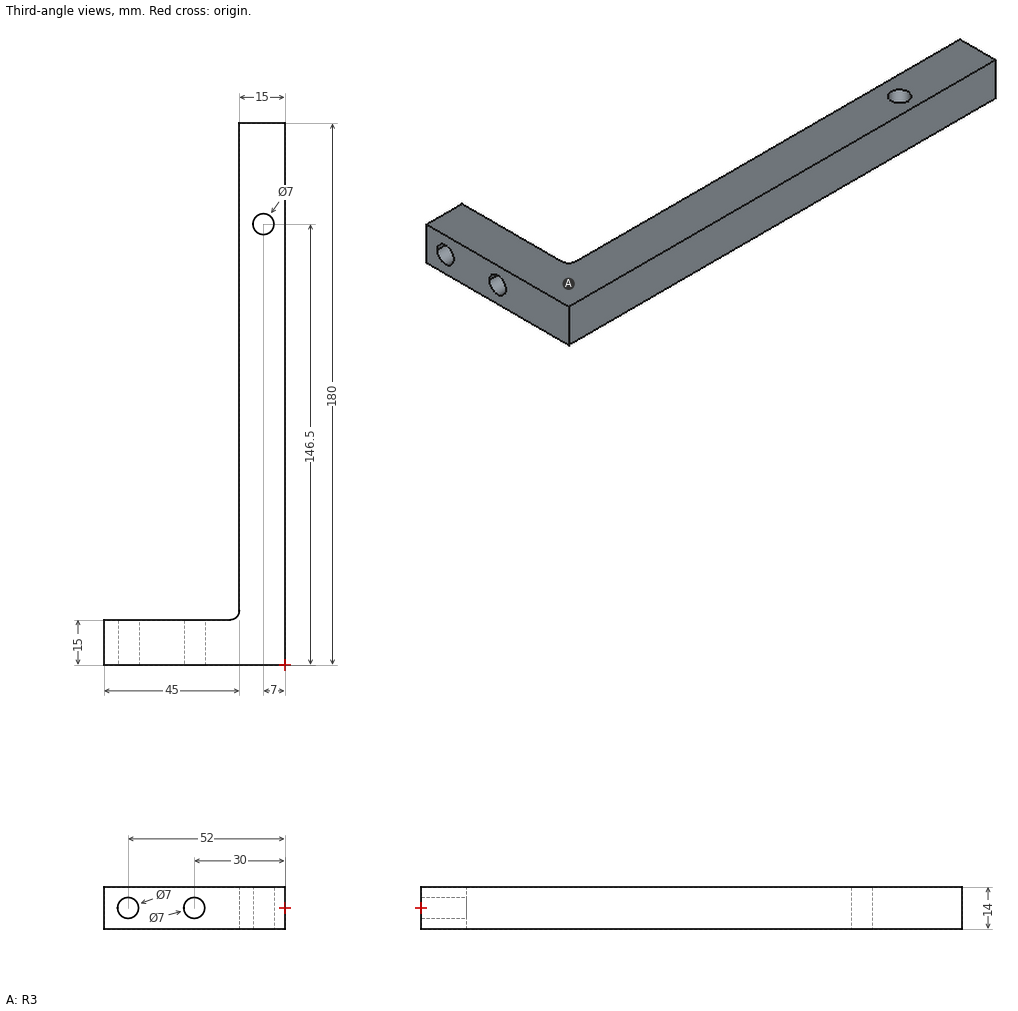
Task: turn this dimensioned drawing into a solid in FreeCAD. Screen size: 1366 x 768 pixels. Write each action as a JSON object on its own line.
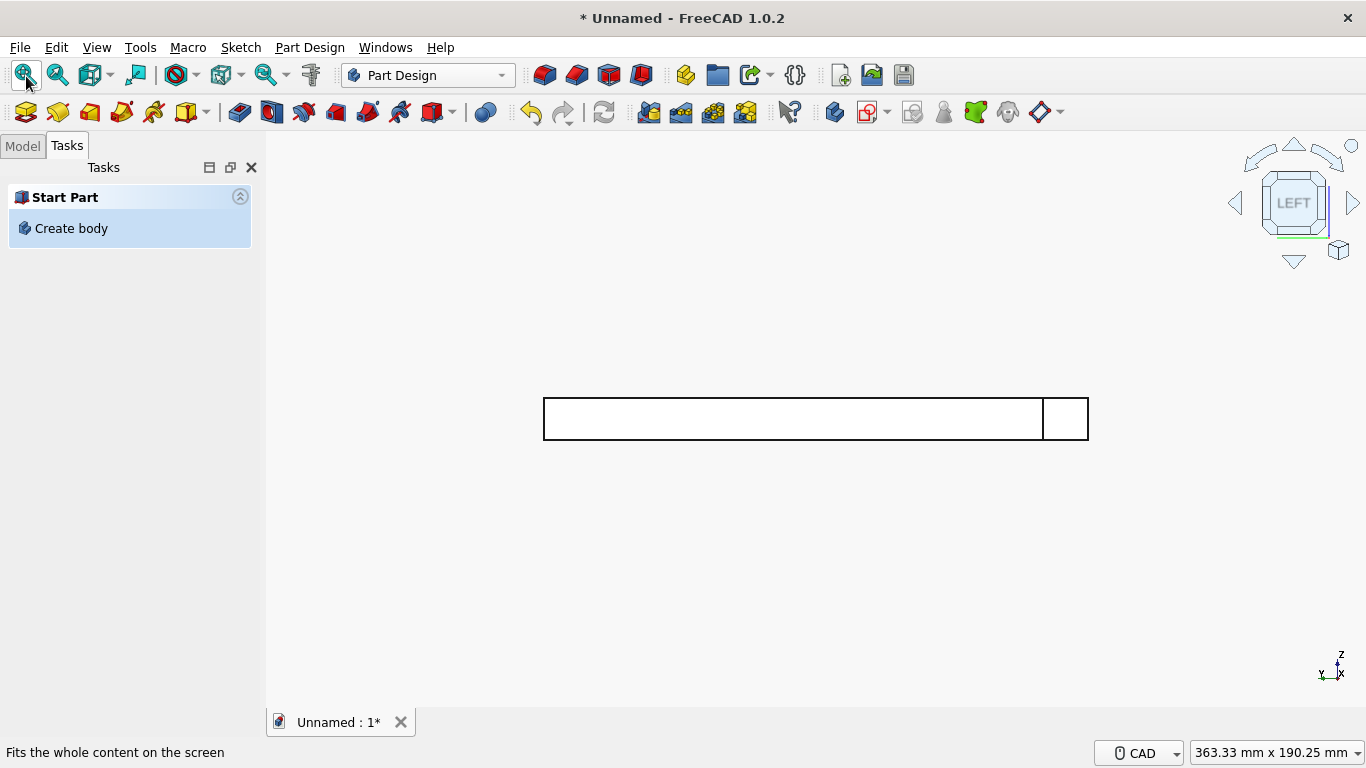
{"action": "key", "text": "v 3"}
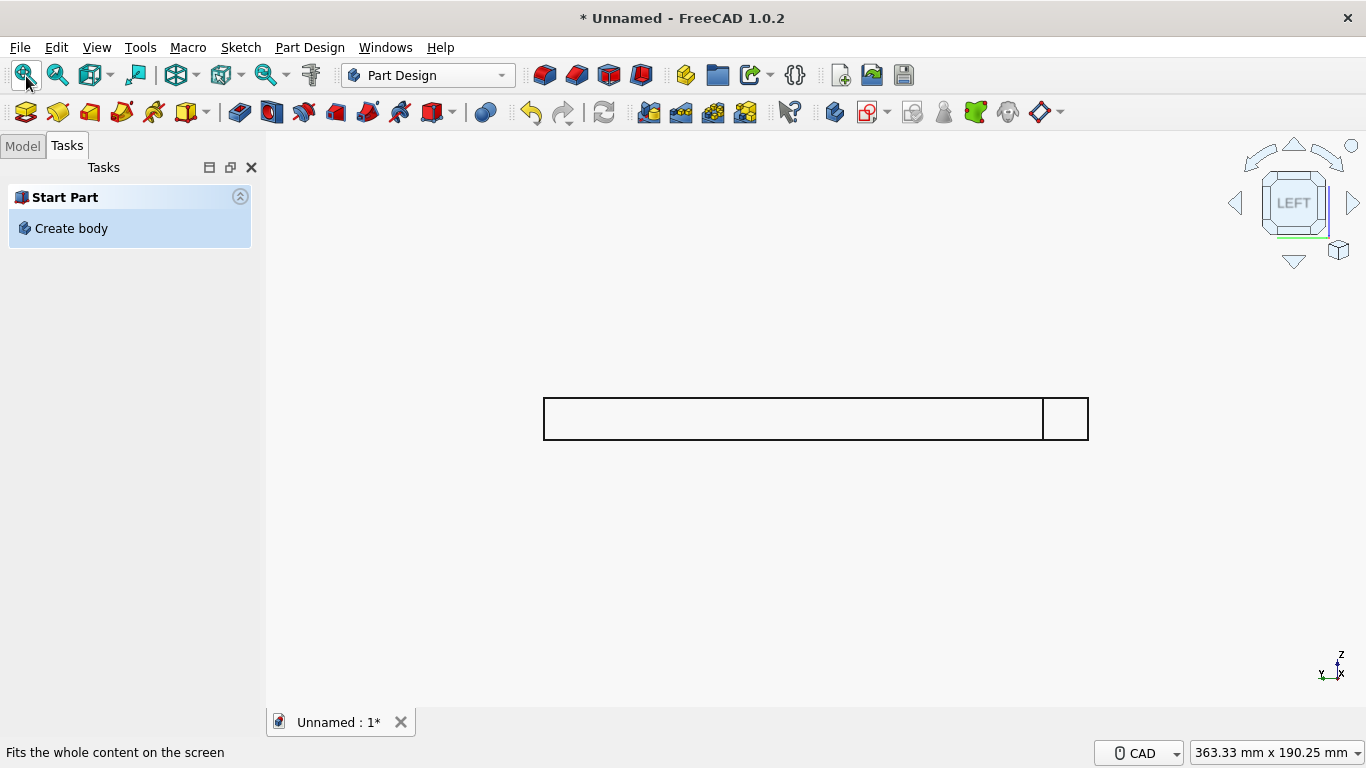
{"action": "key", "text": "0"}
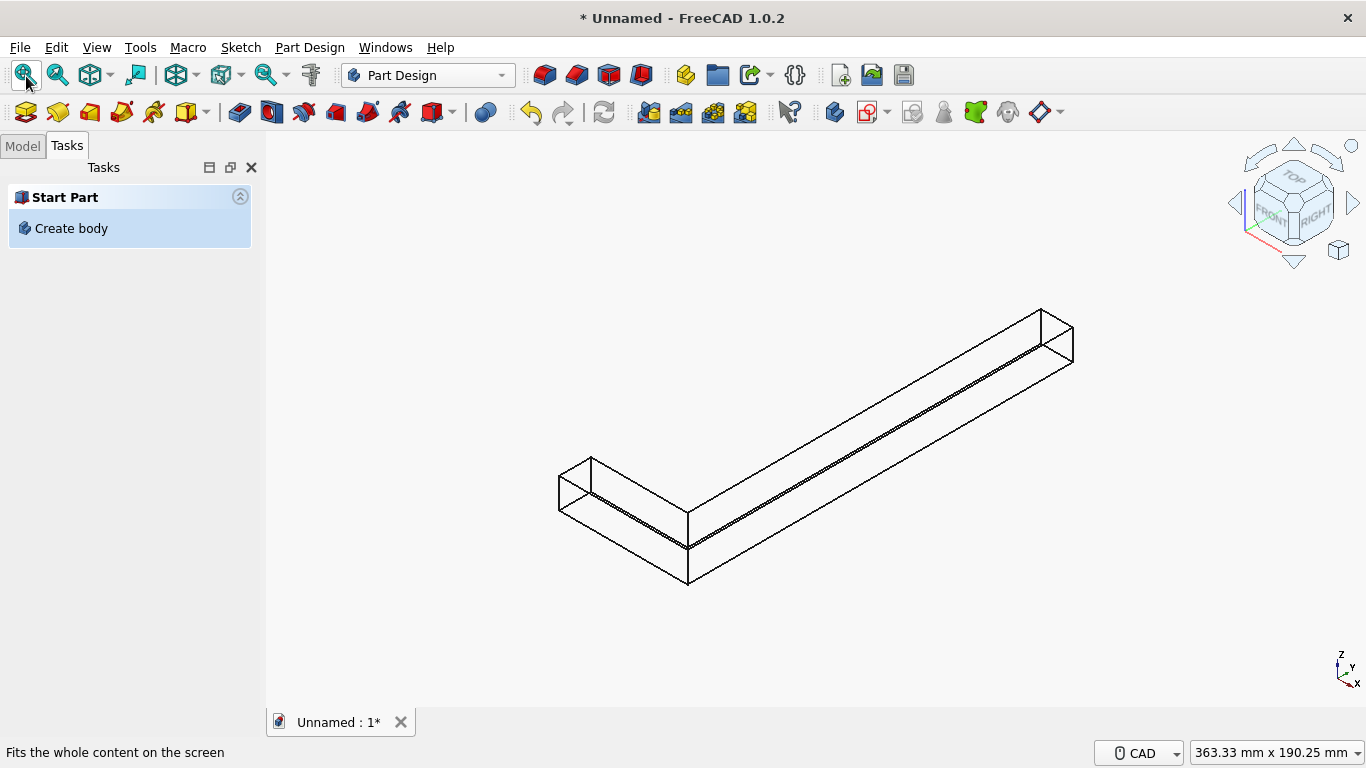
{"action": "left_click", "coordinate": [688, 529]}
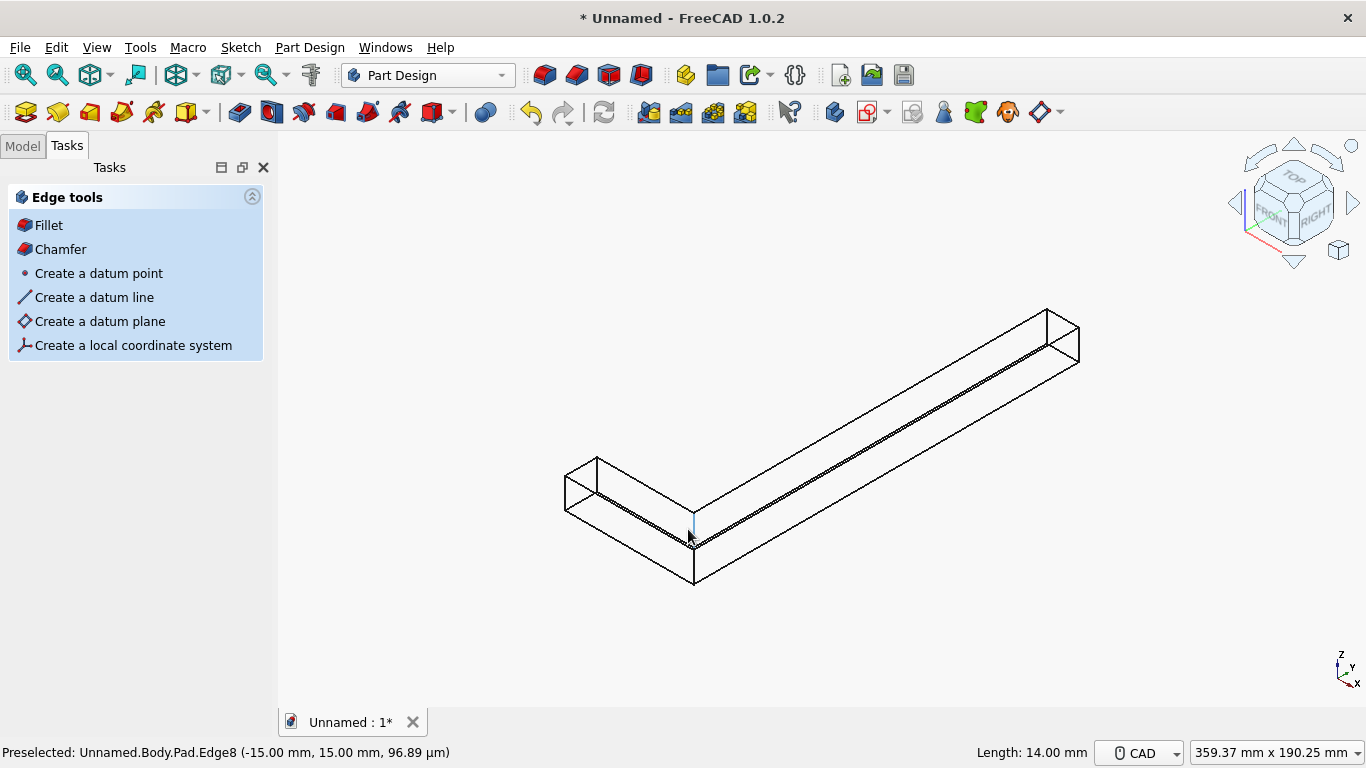
{"action": "key", "text": "v 1"}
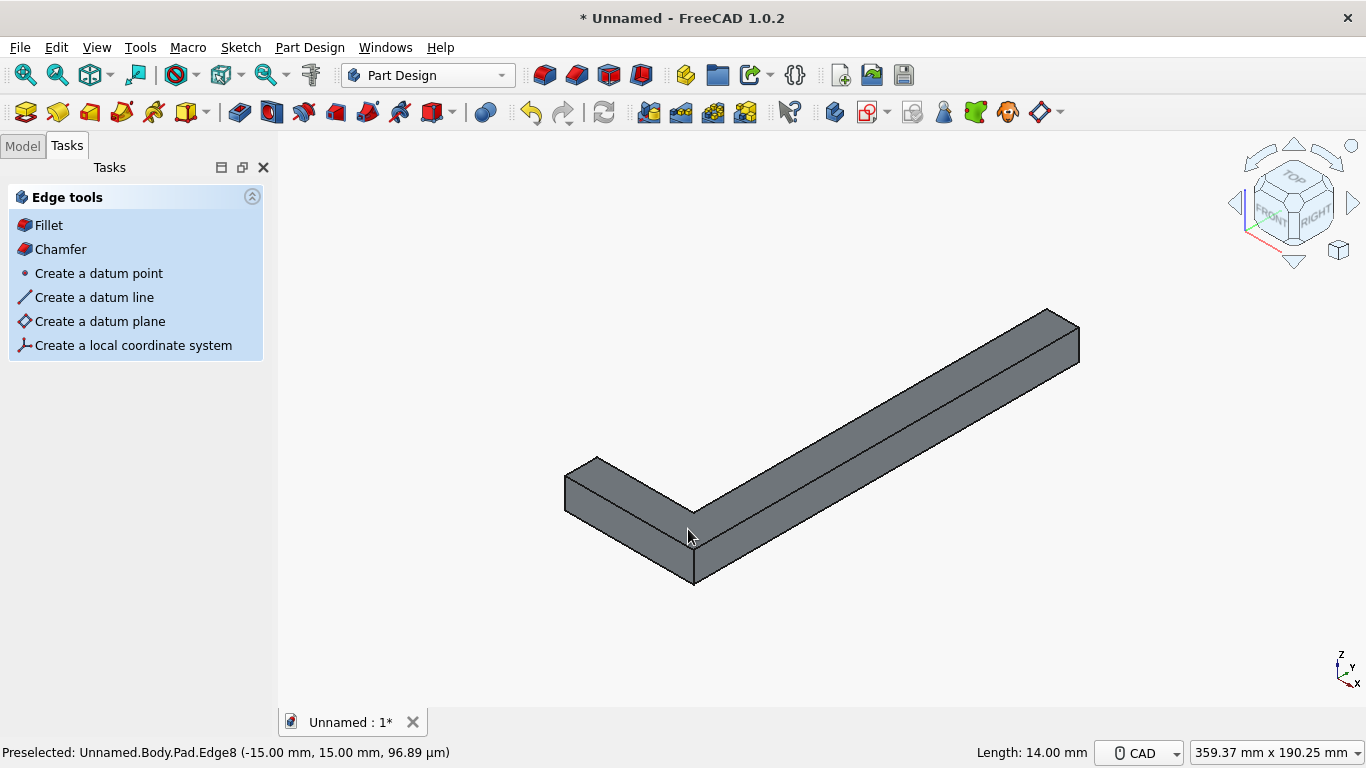
{"action": "left_click", "coordinate": [546, 76]}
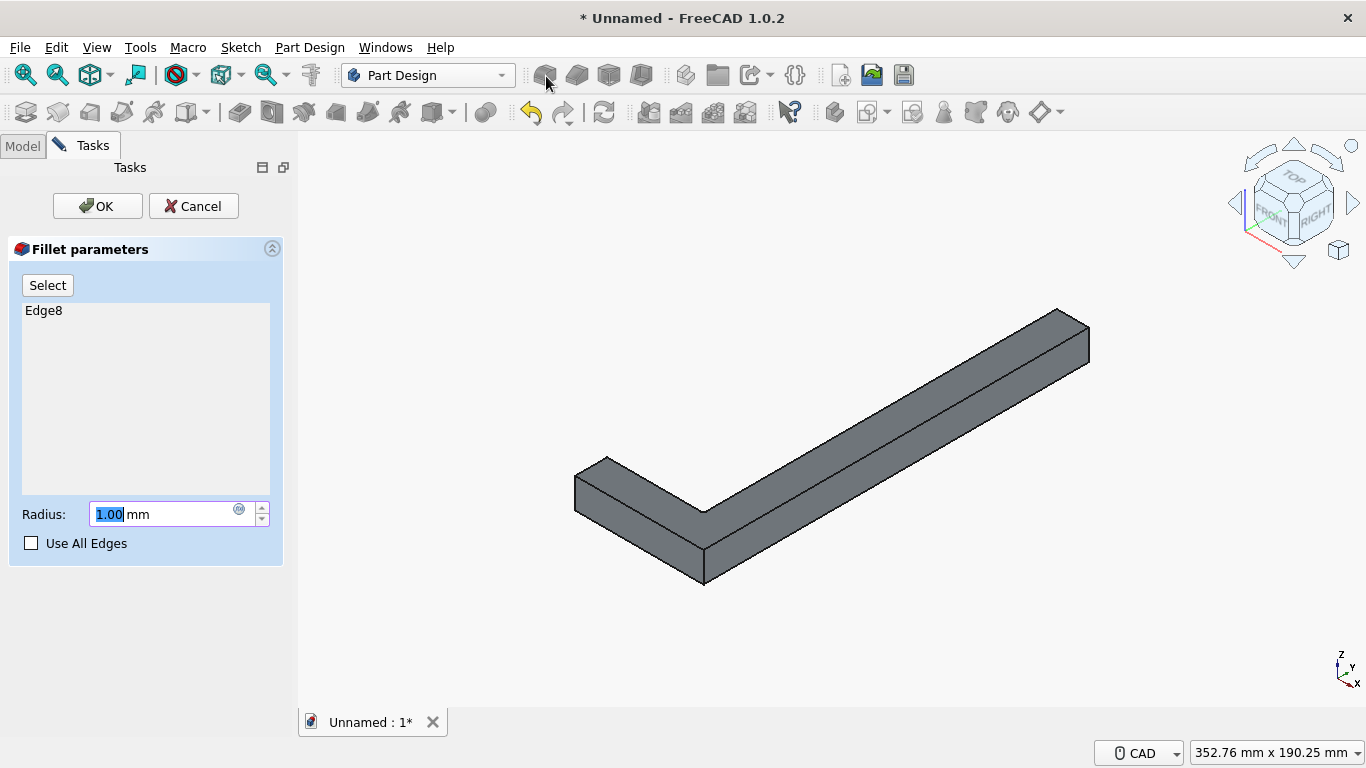
{"action": "type", "text": "3"}
{"action": "key", "text": "Tab"}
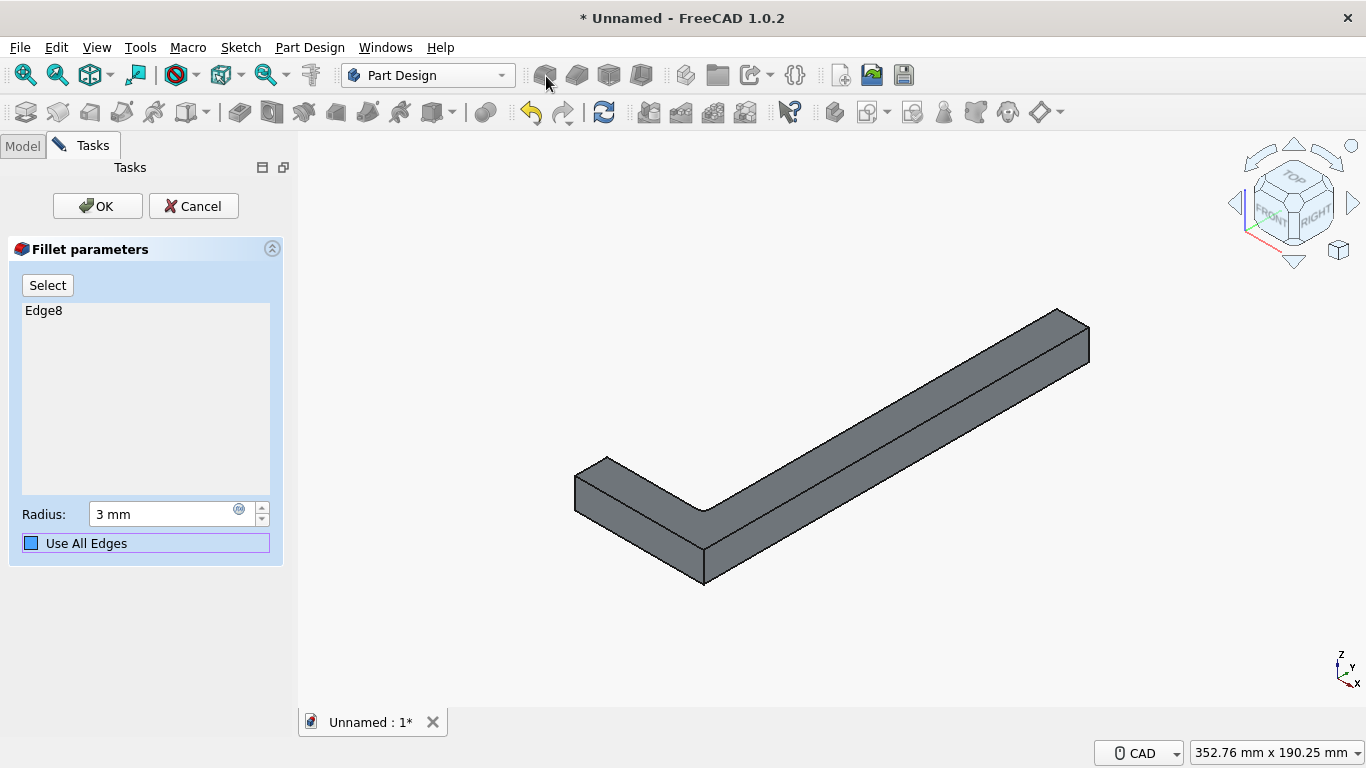
{"action": "left_click", "coordinate": [98, 206]}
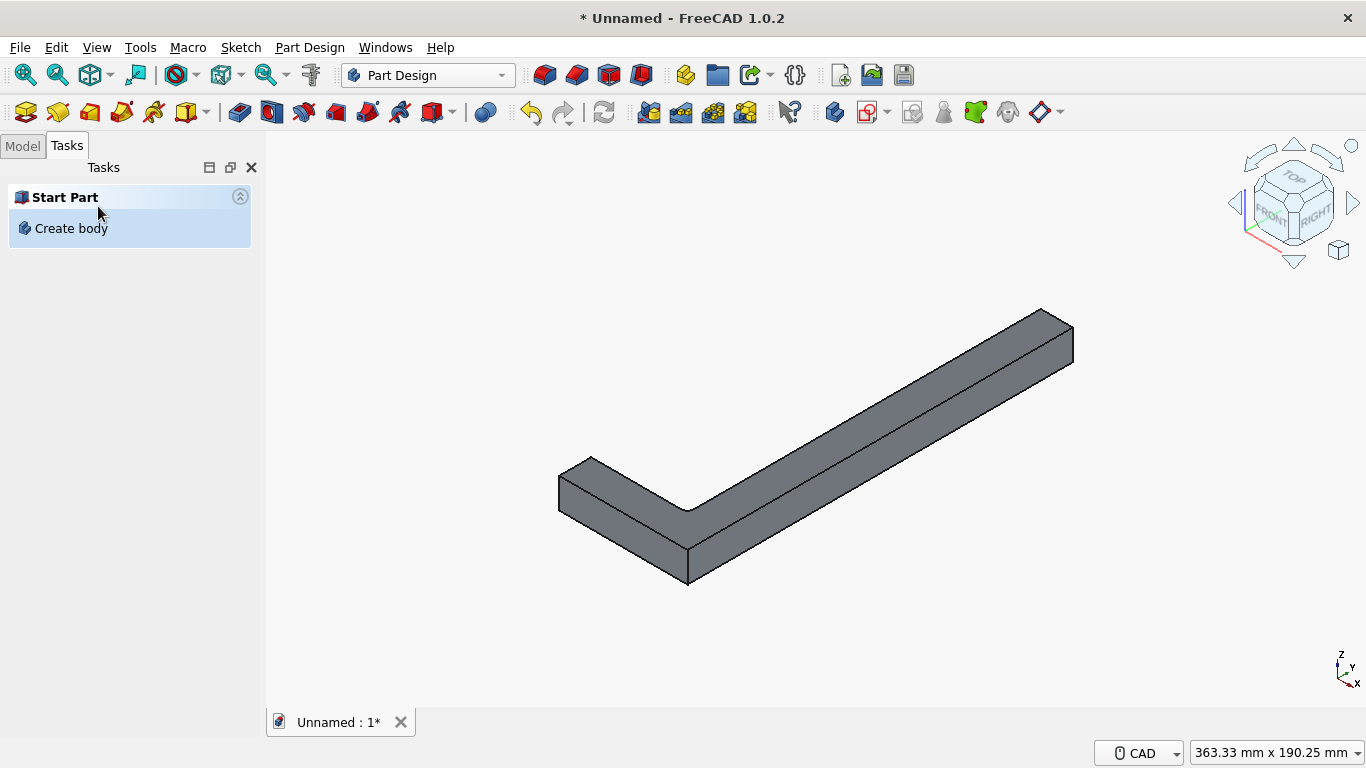
{"action": "key", "text": "4"}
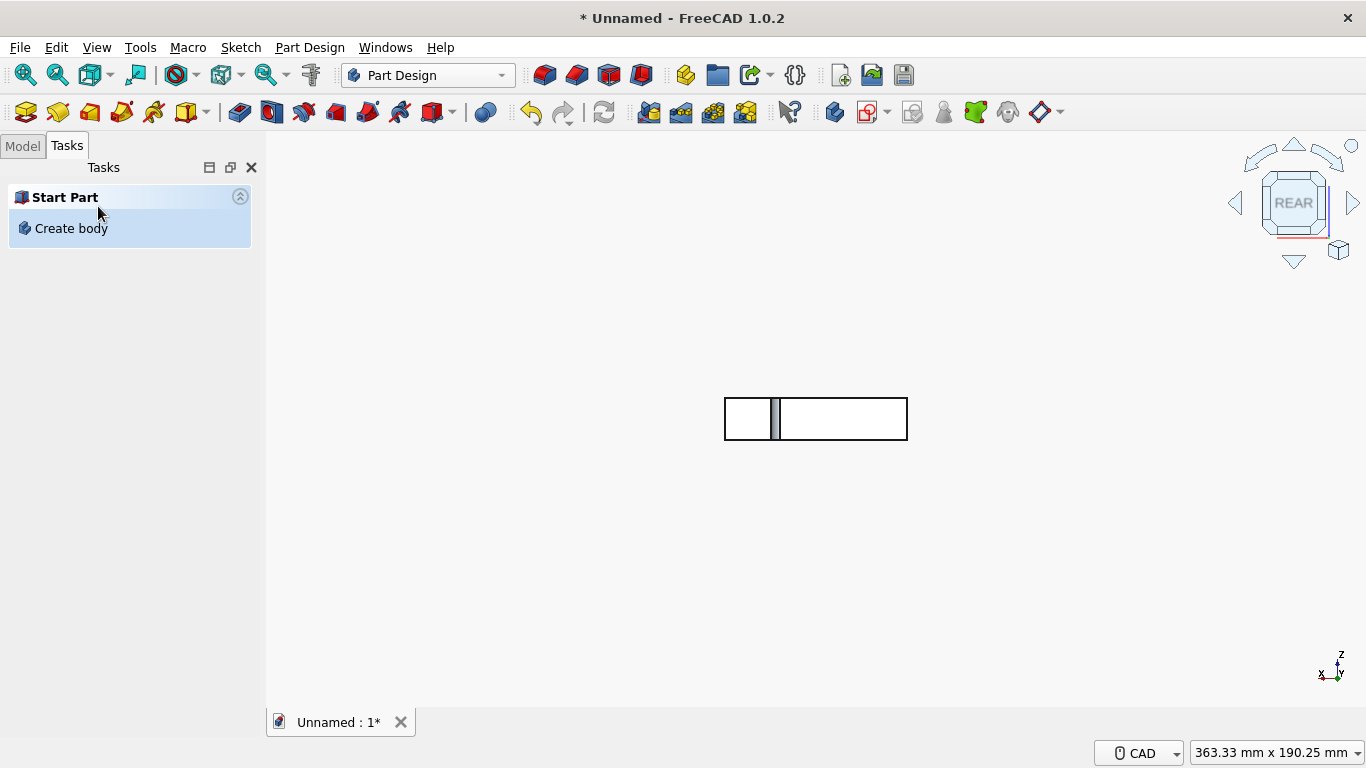
{"action": "left_click", "coordinate": [26, 76]}